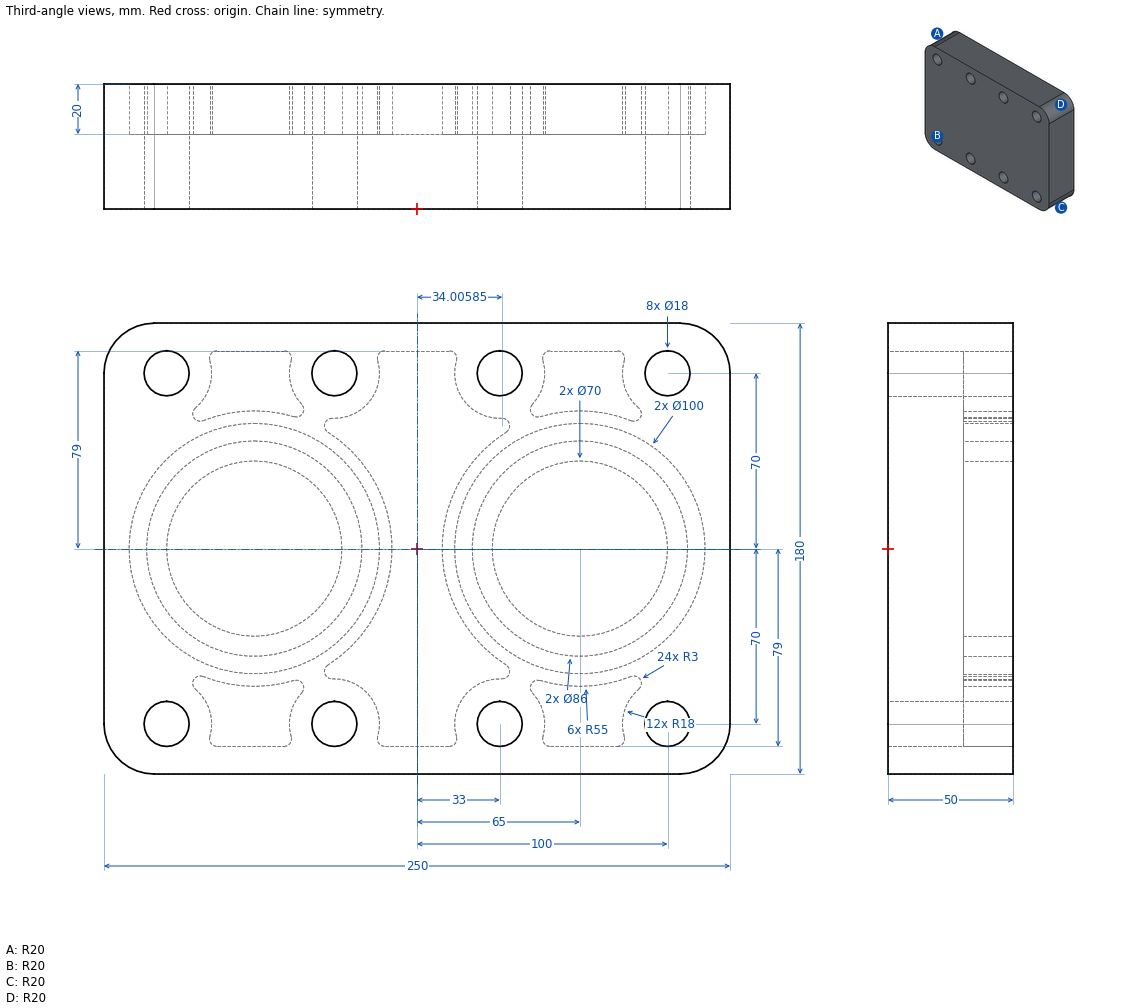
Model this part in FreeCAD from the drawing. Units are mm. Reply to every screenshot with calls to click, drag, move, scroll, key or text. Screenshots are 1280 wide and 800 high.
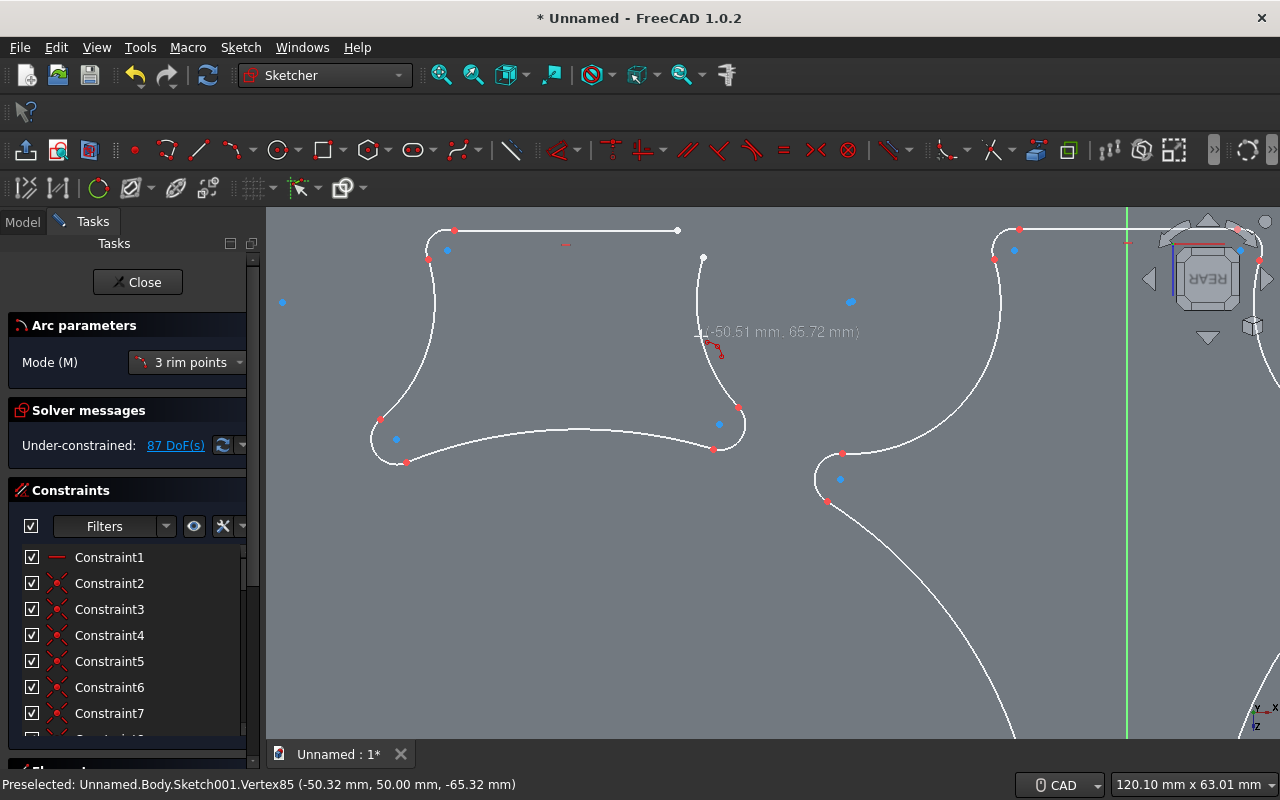
click(703, 258)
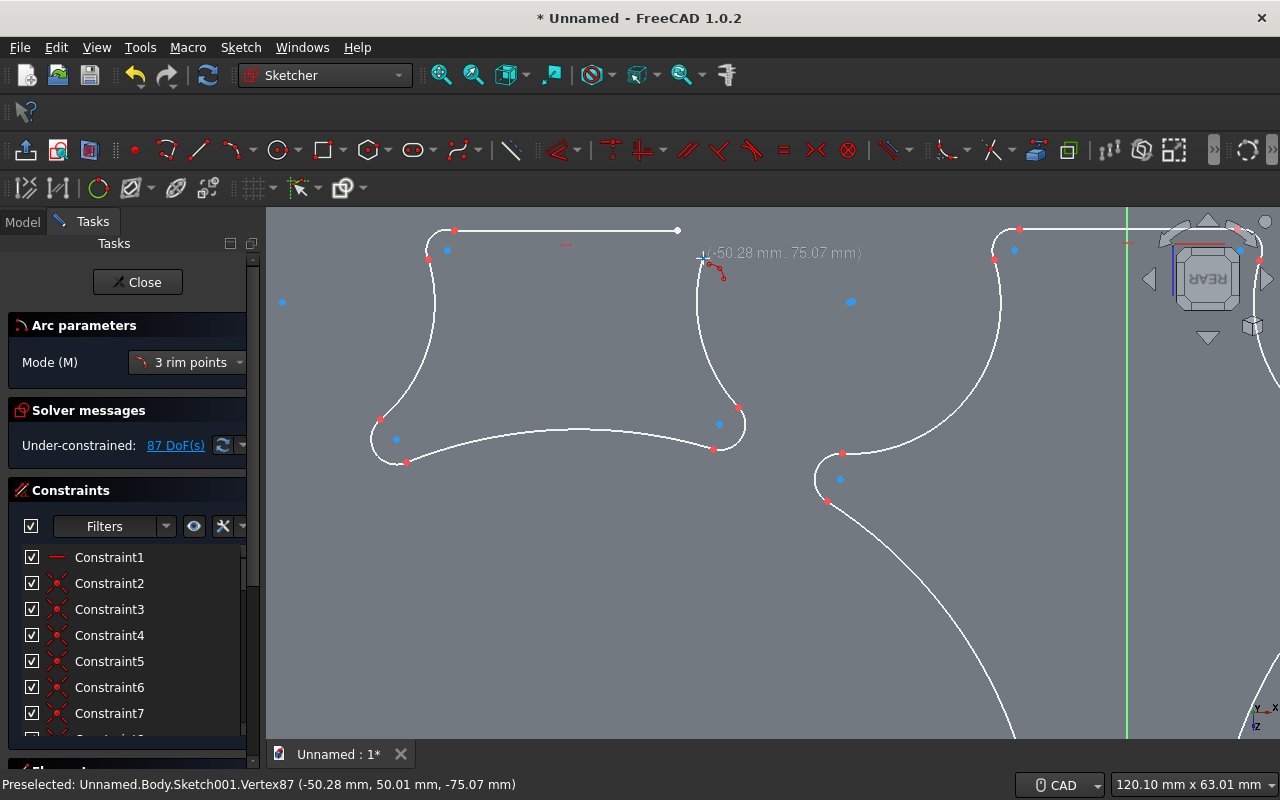
scroll(566, 336, down, 7)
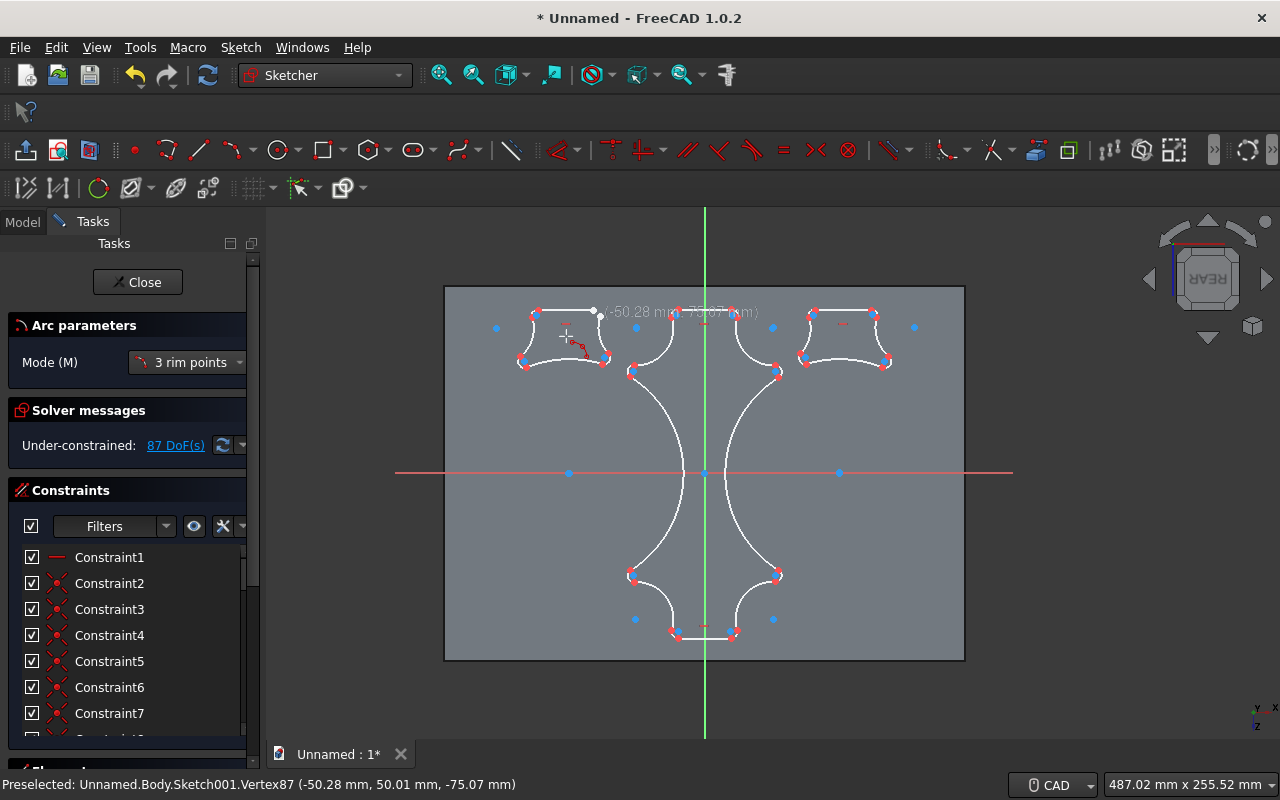
scroll(594, 309, up, 3)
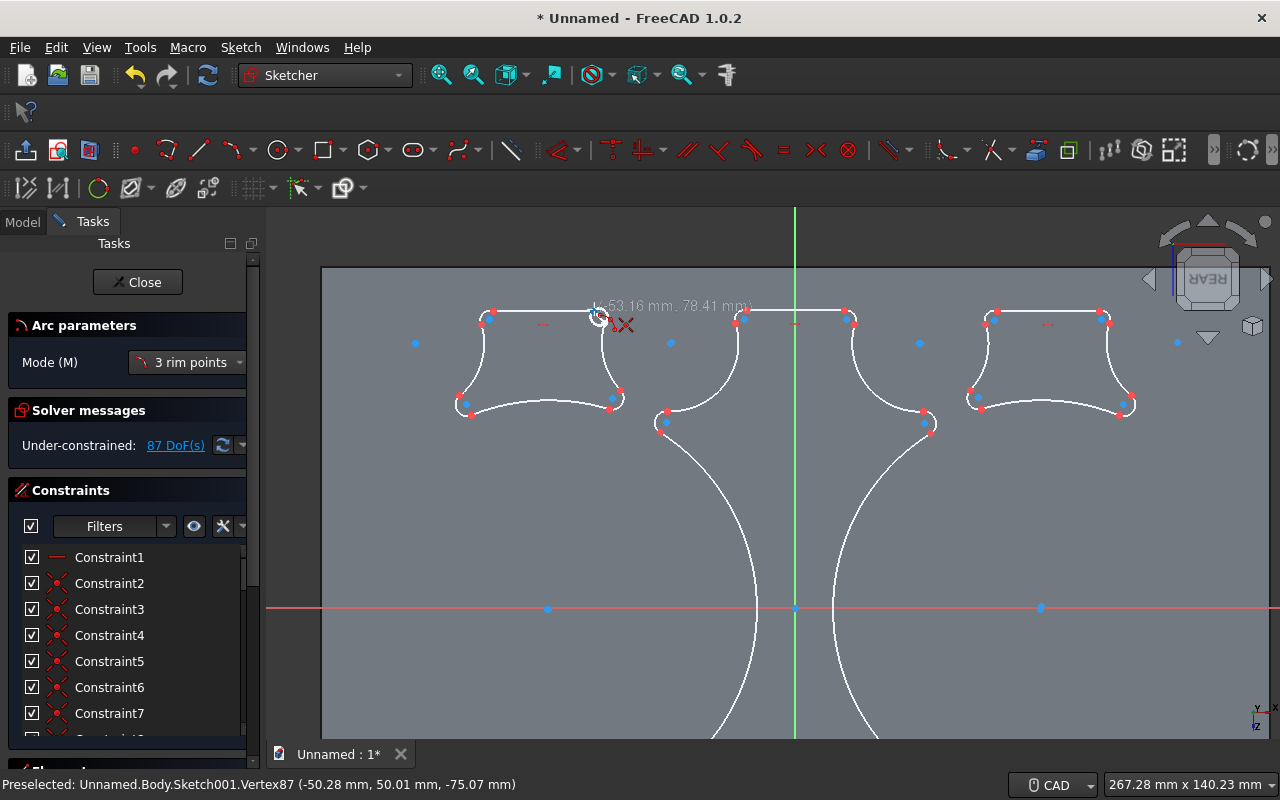
click(593, 311)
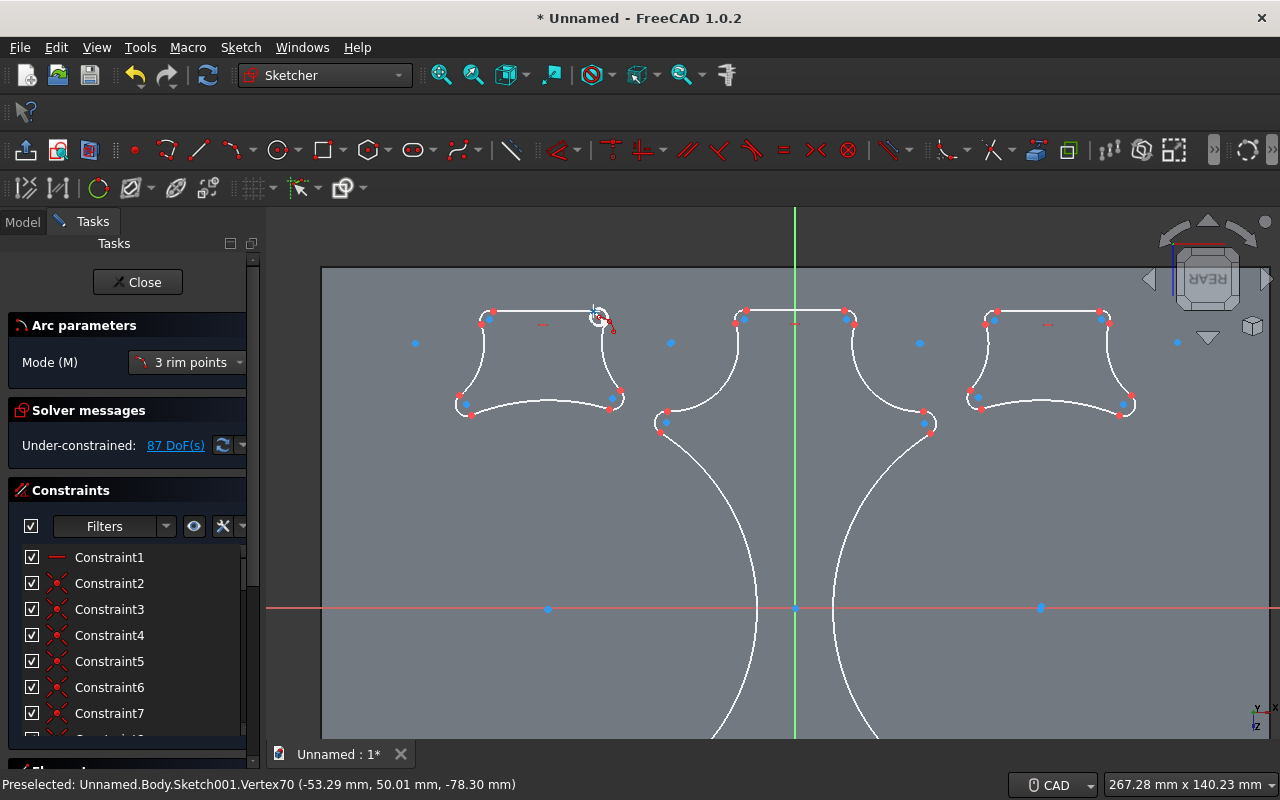
scroll(603, 313, up, 7)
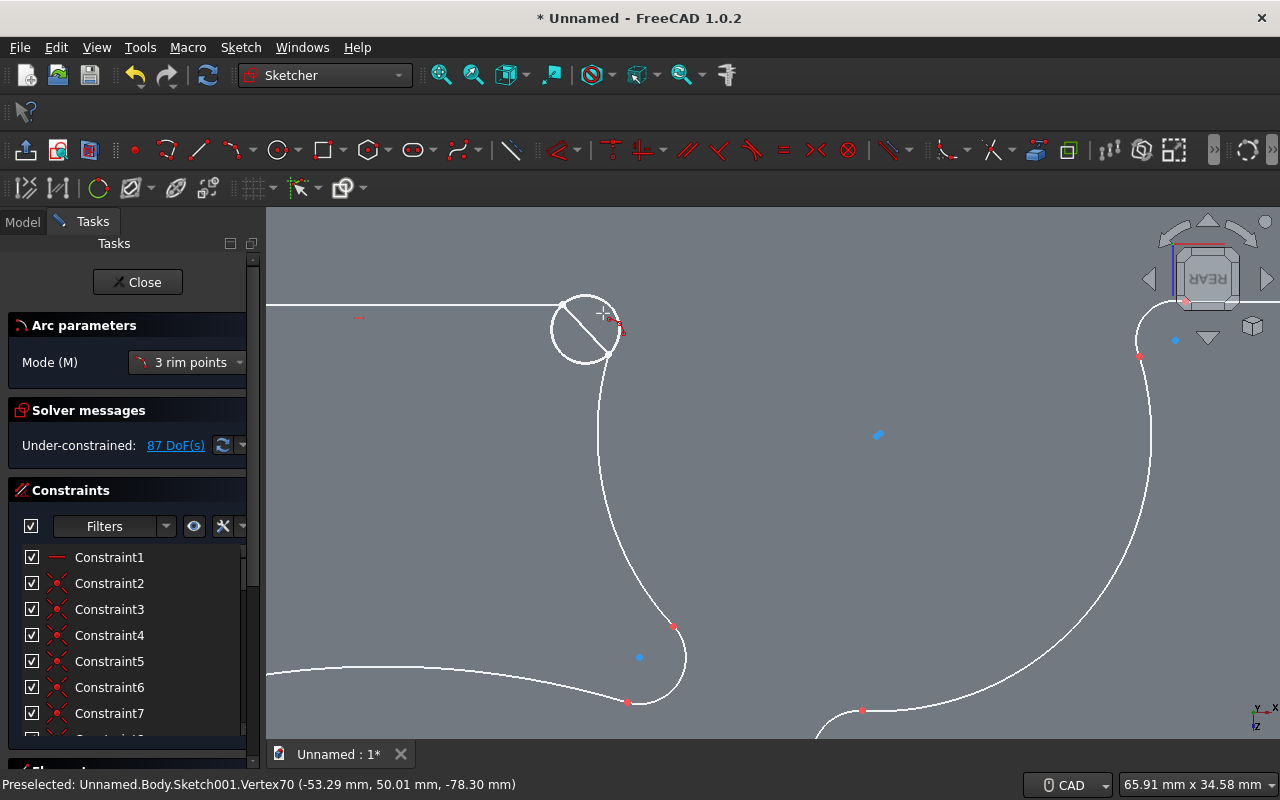
click(602, 312)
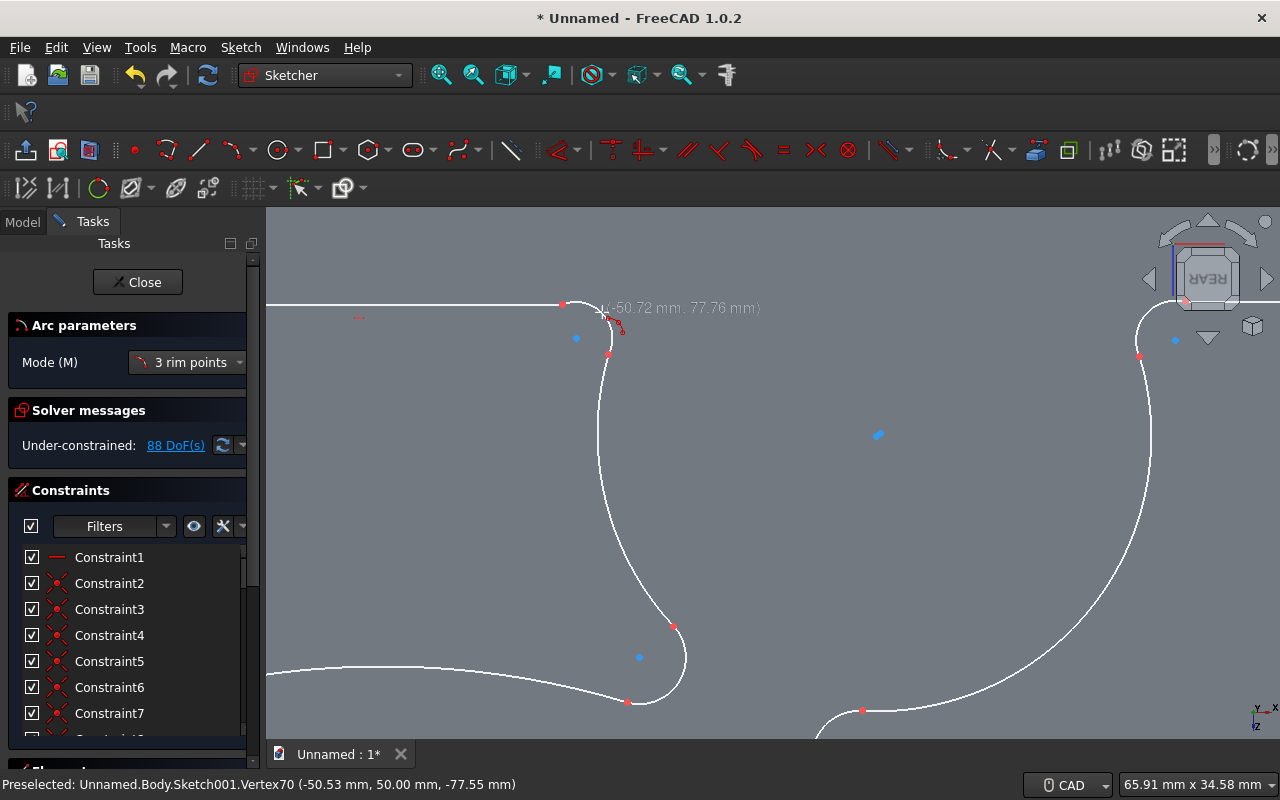
click(200, 150)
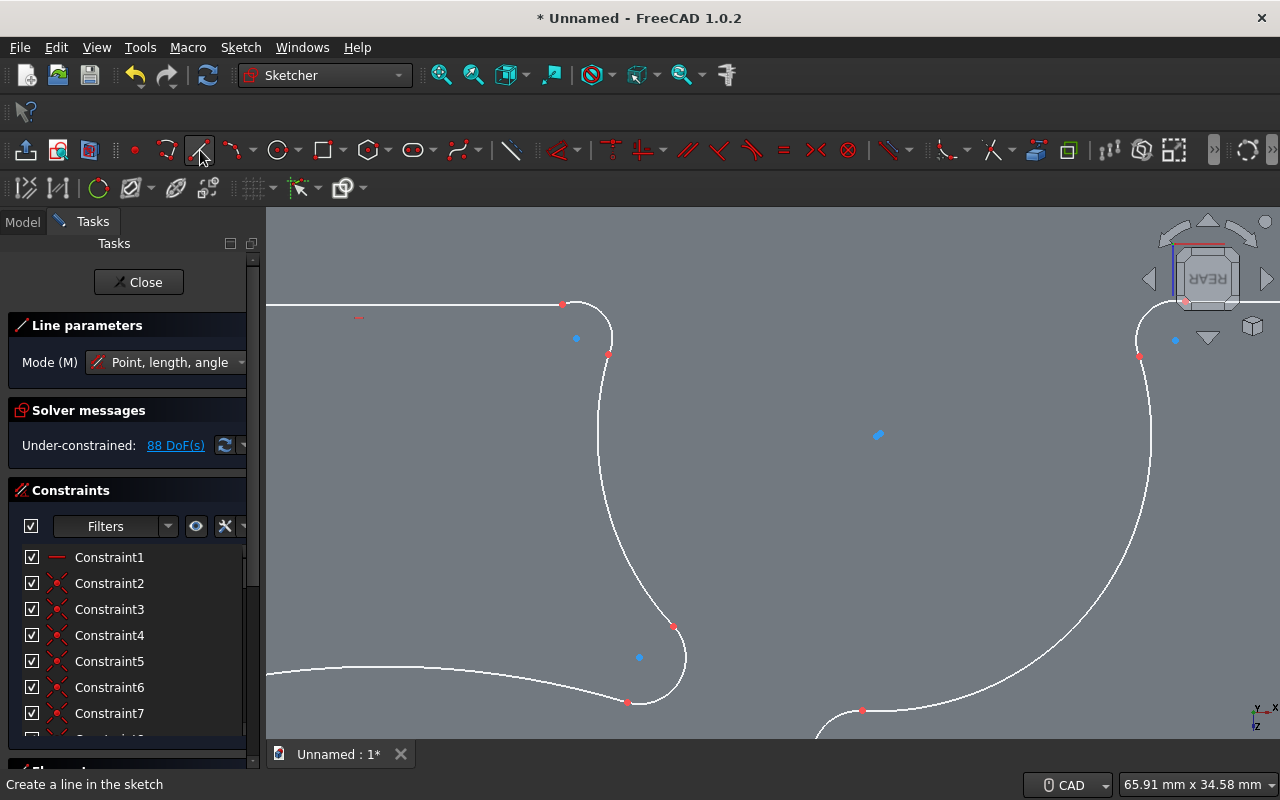
scroll(598, 311, down, 10)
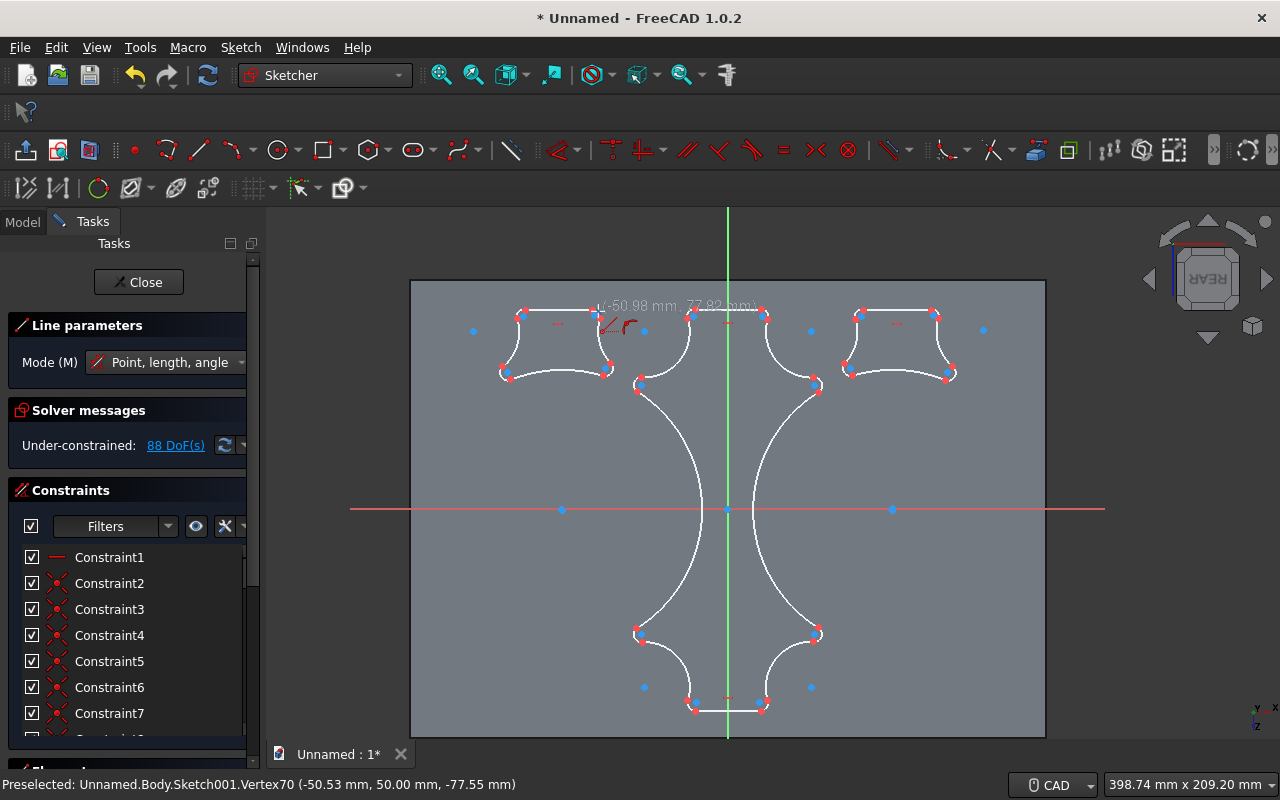
click(538, 638)
click(594, 638)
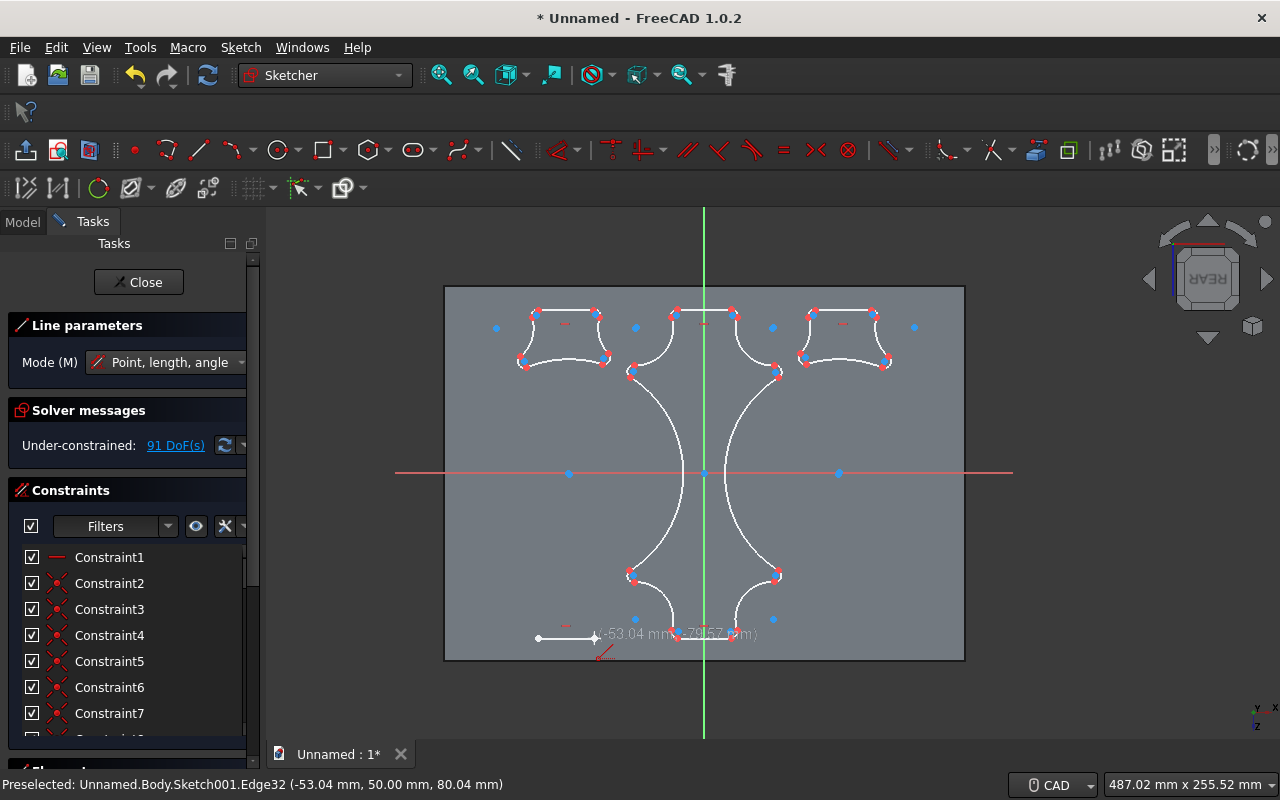
click(232, 150)